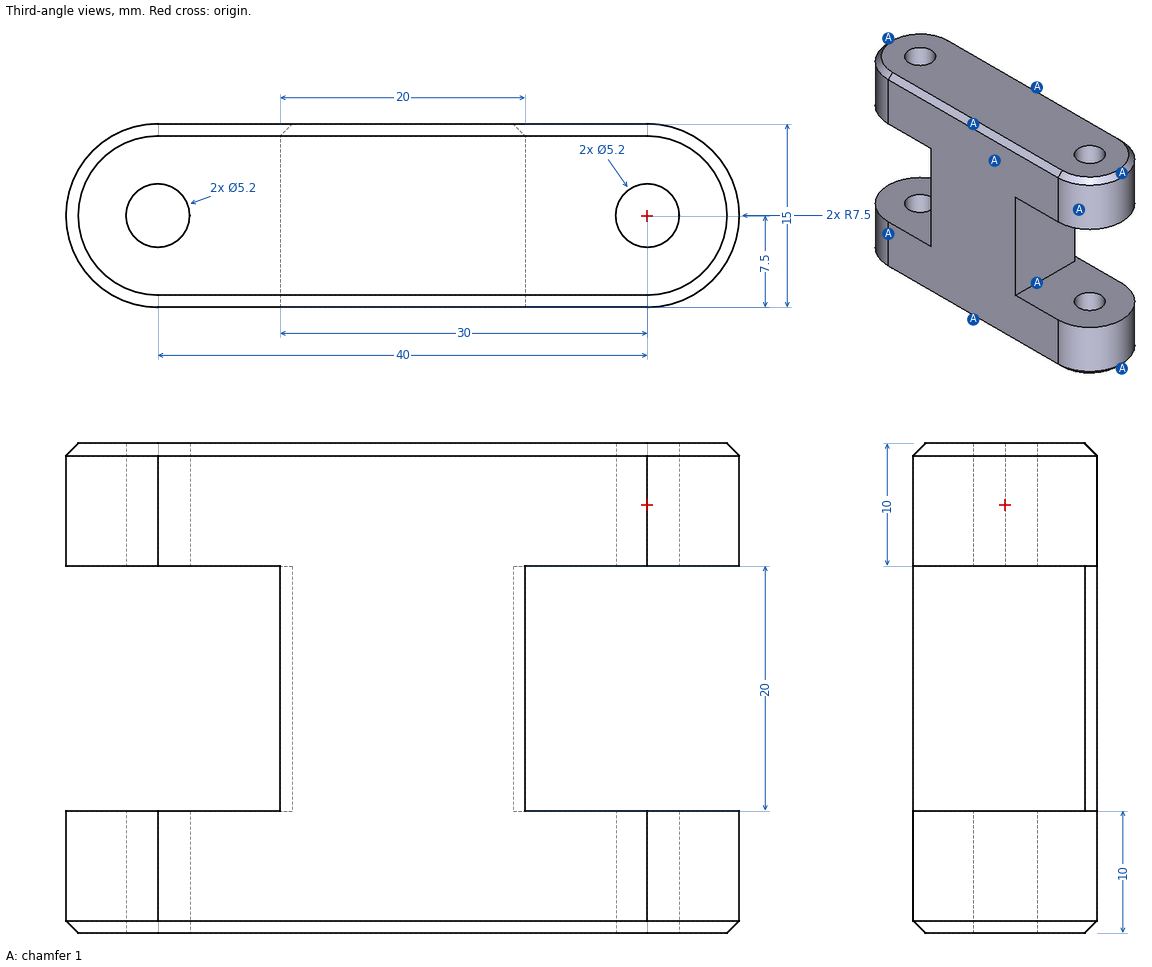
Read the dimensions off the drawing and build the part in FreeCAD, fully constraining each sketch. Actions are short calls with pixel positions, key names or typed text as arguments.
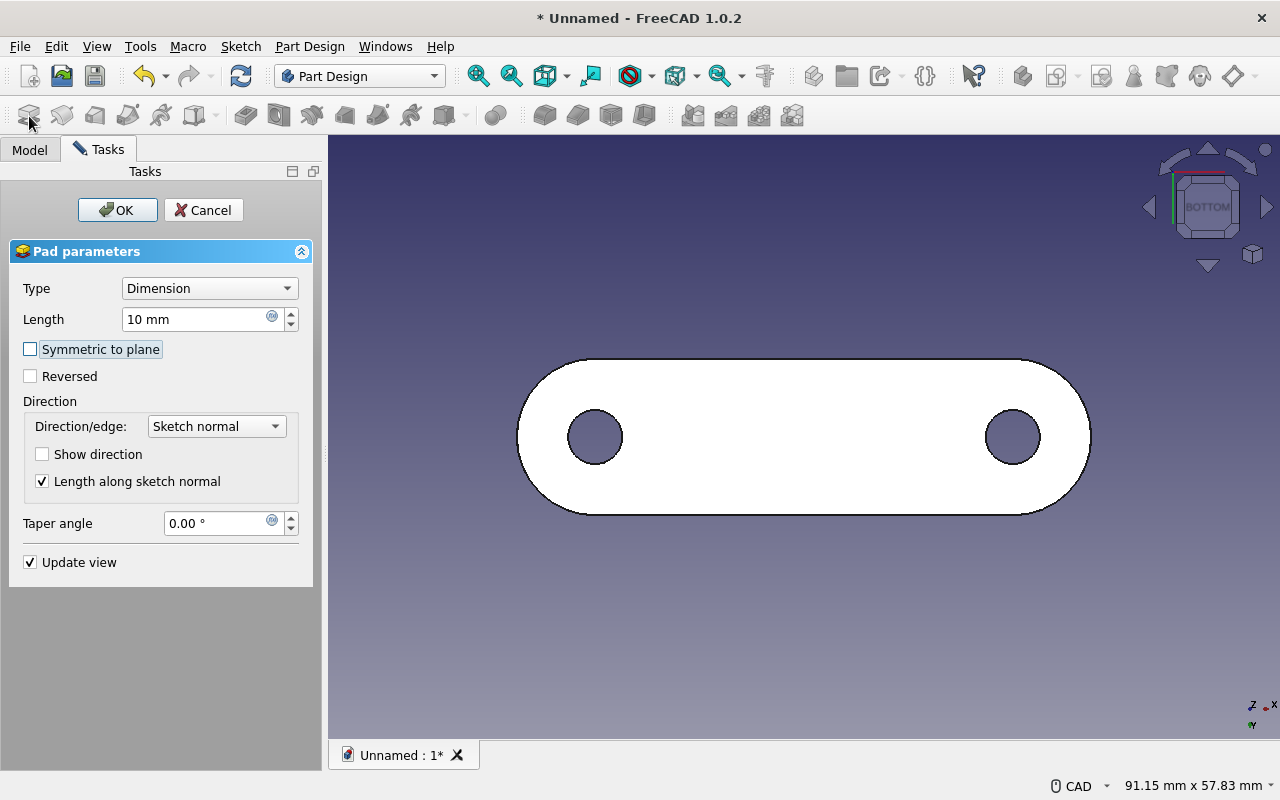
click(118, 210)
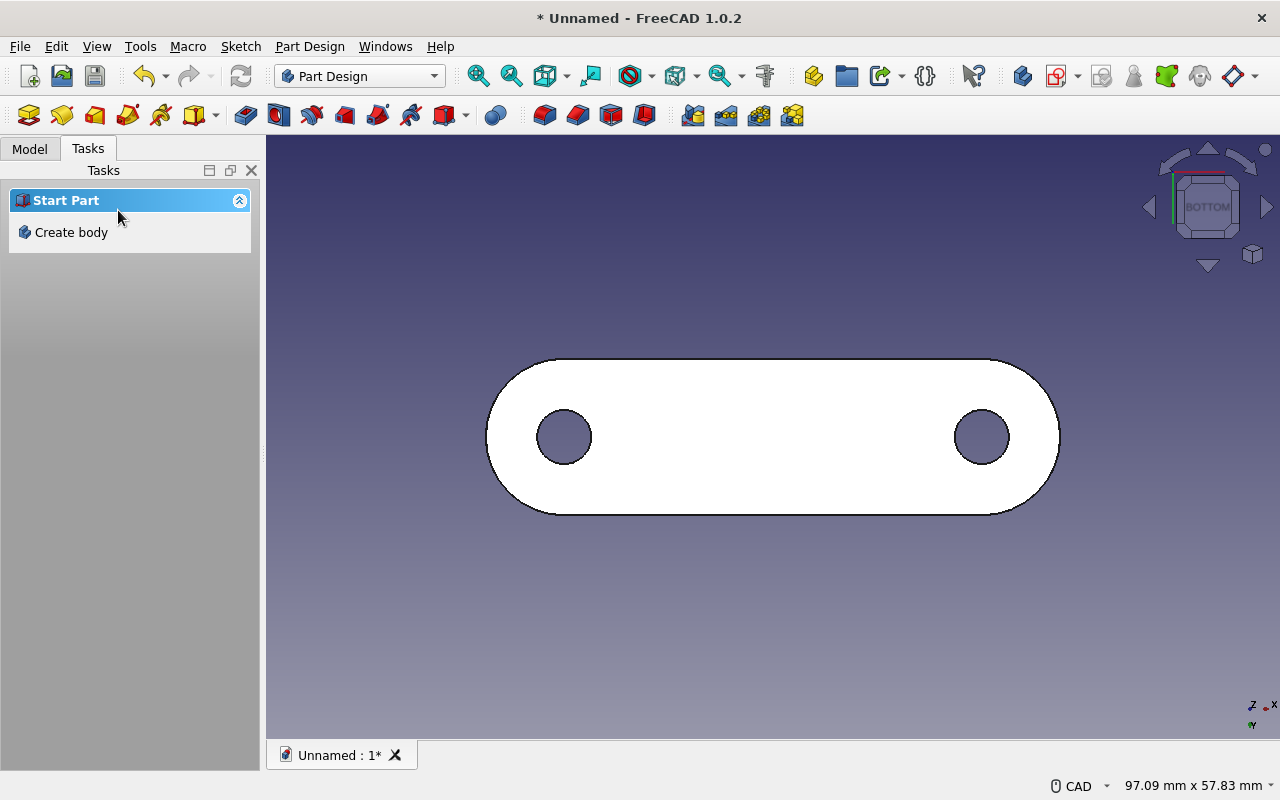
click(1060, 436)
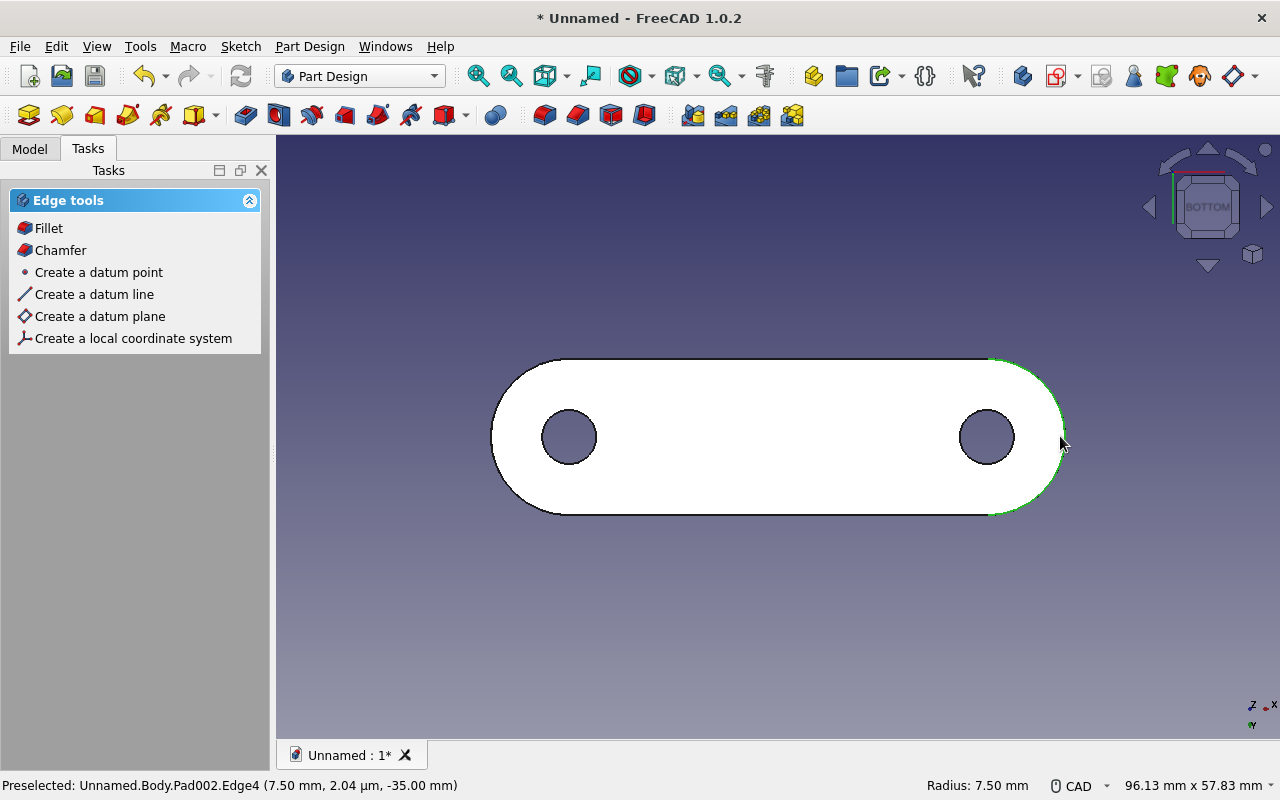
click(491, 436, ctrl)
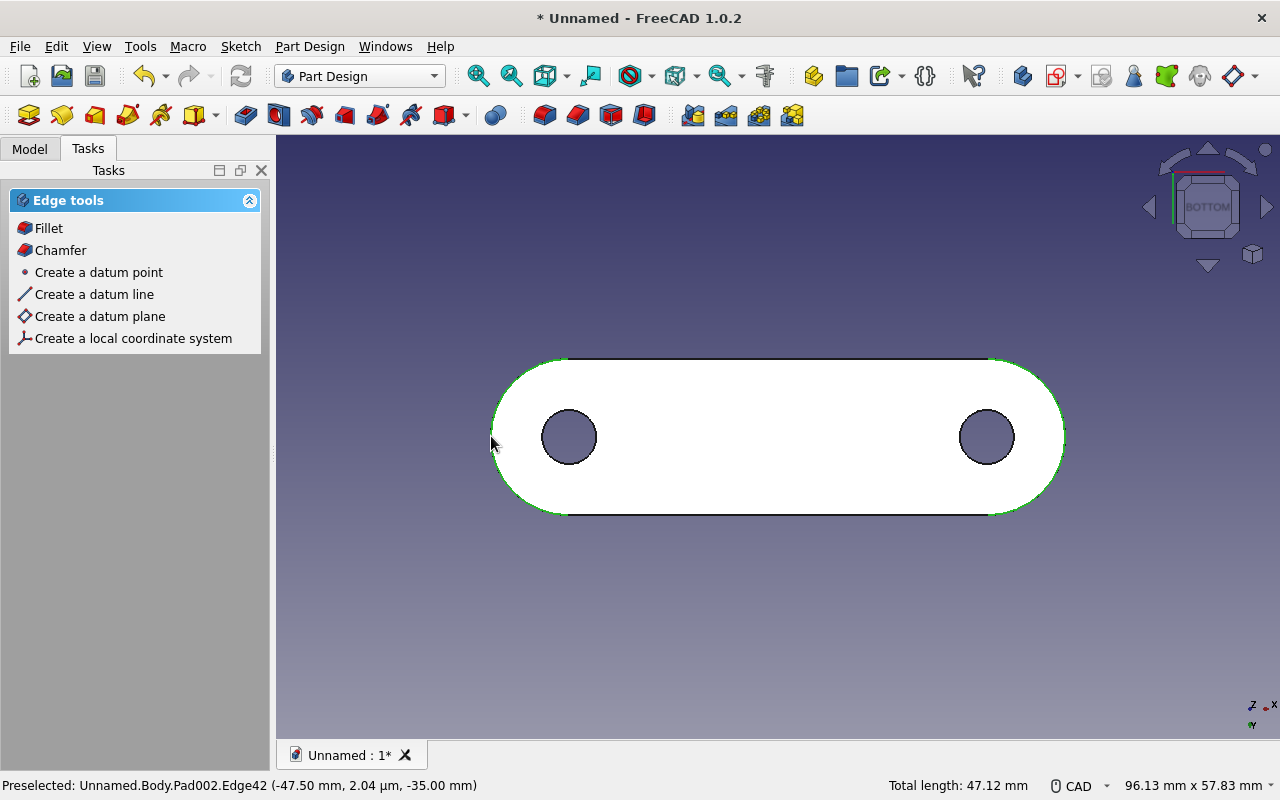
click(778, 514, ctrl)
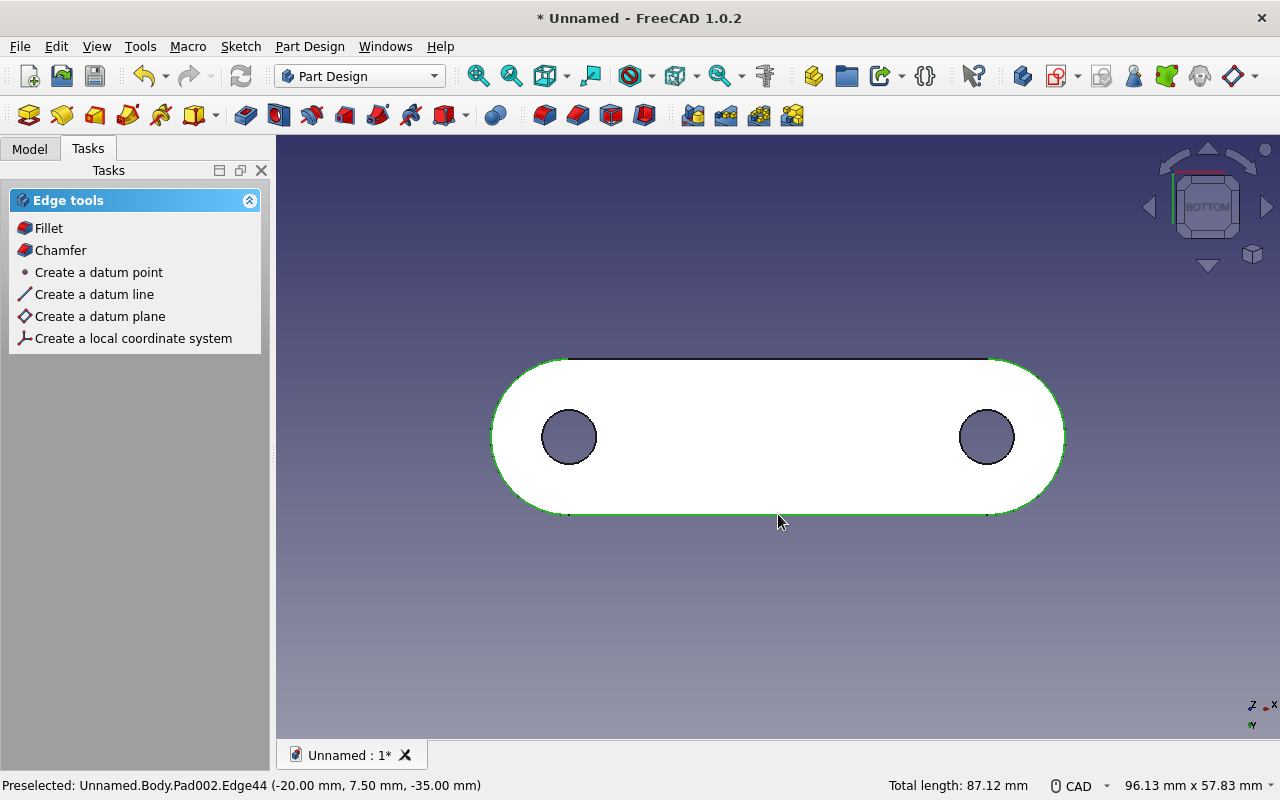
key(0)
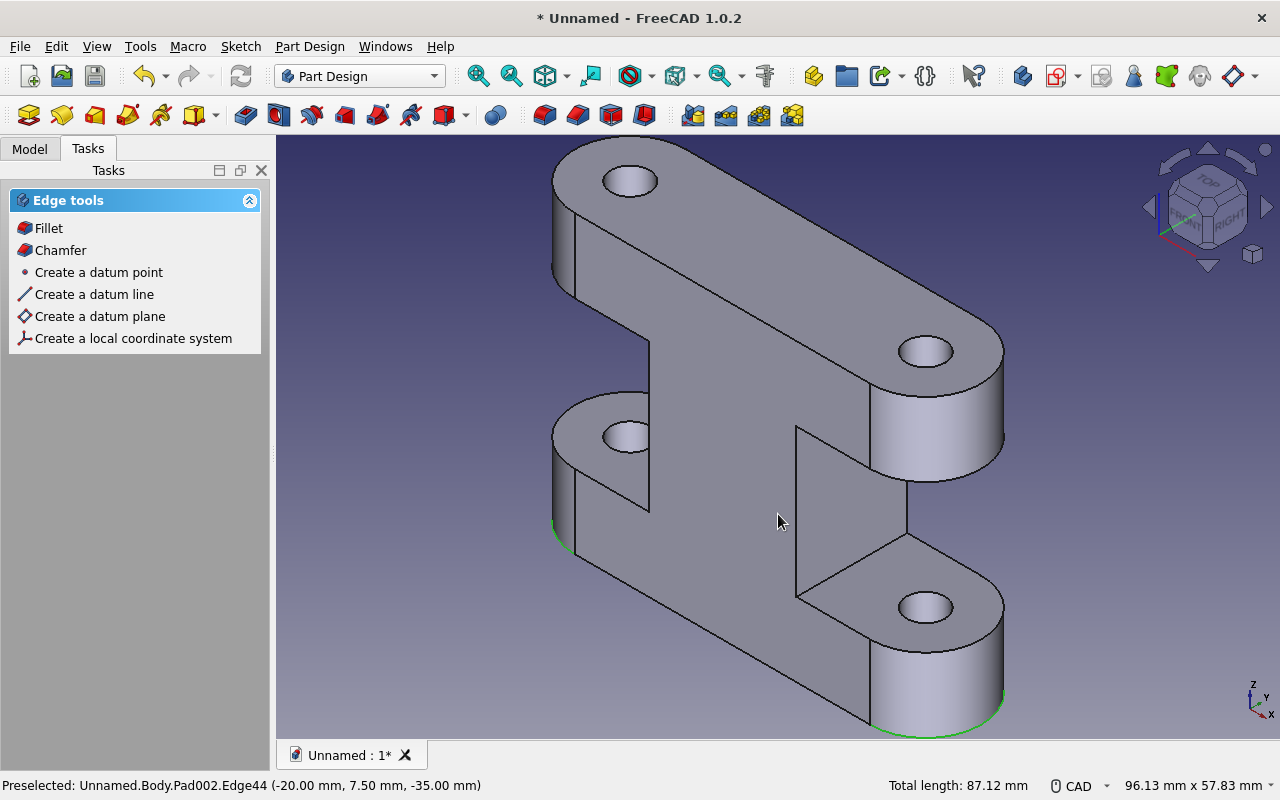
key(v)
key(f)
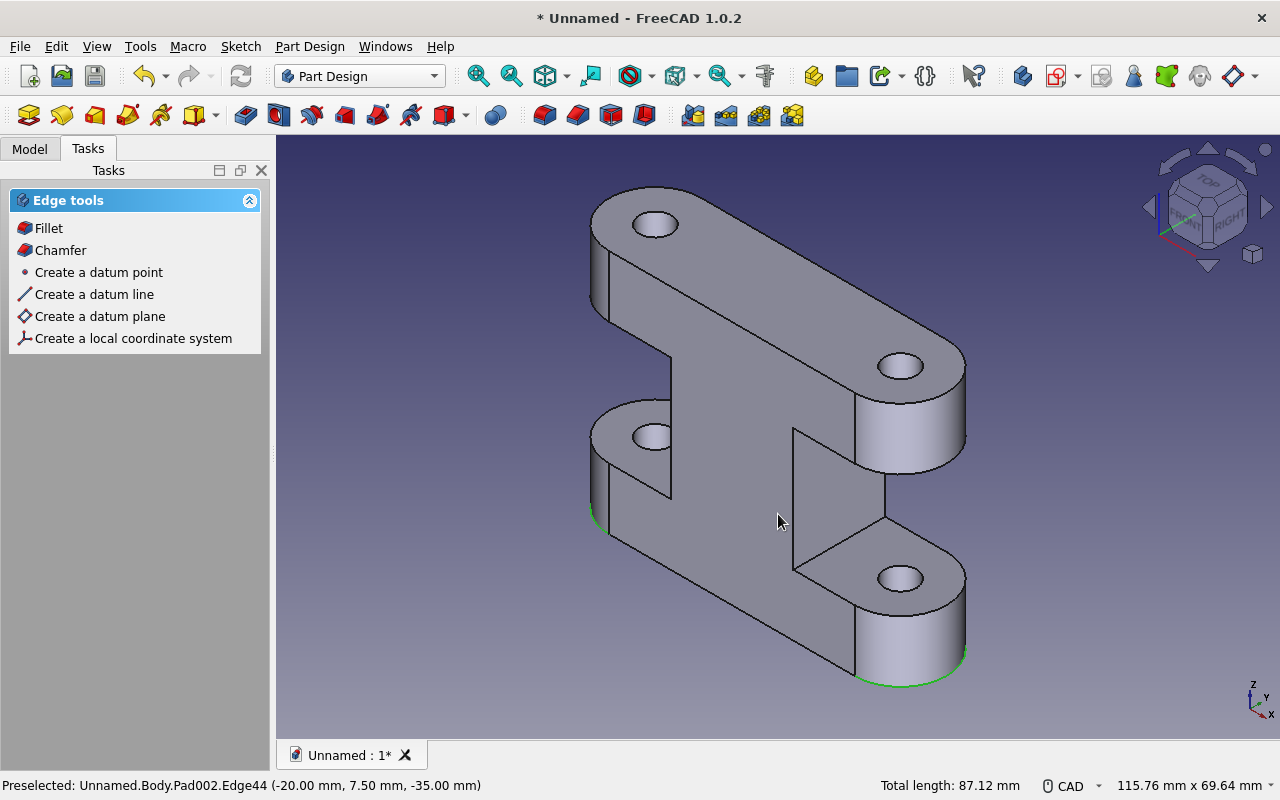
click(591, 229, ctrl)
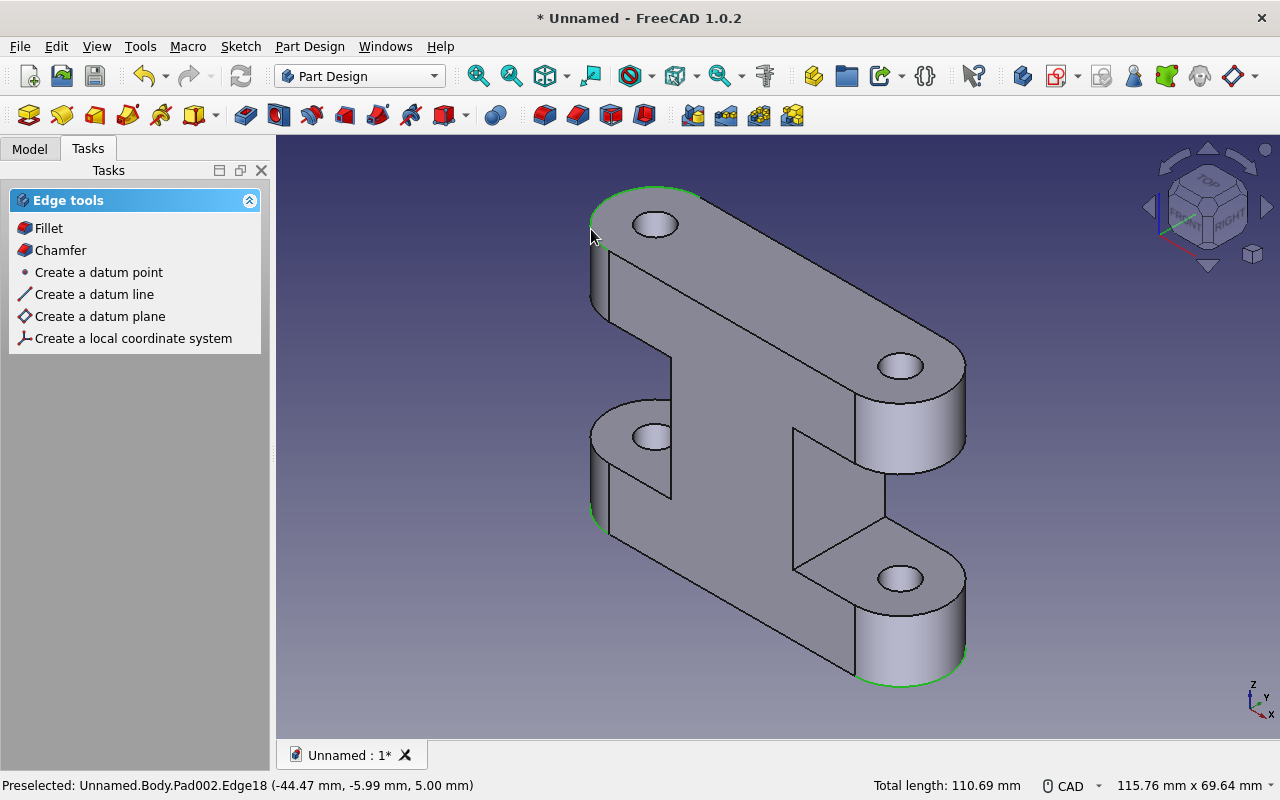
click(732, 321, ctrl)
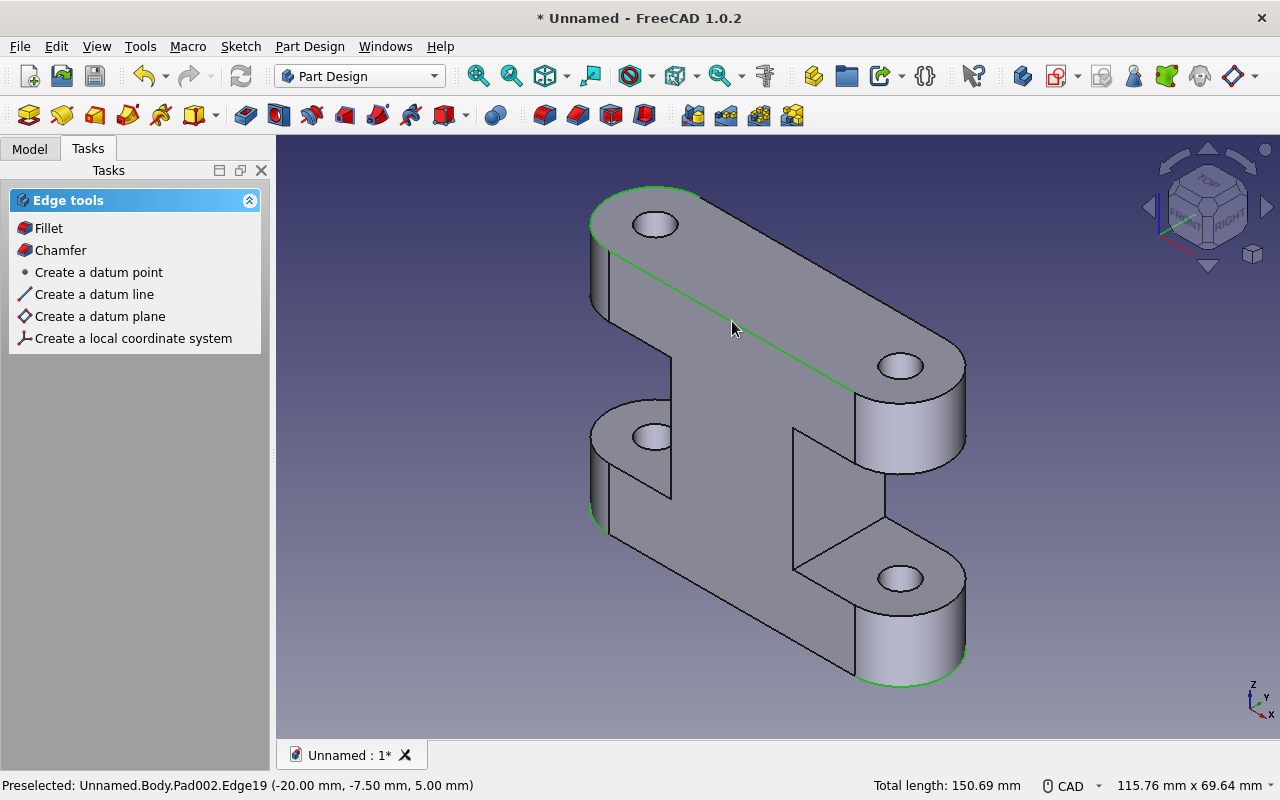
click(947, 392, ctrl)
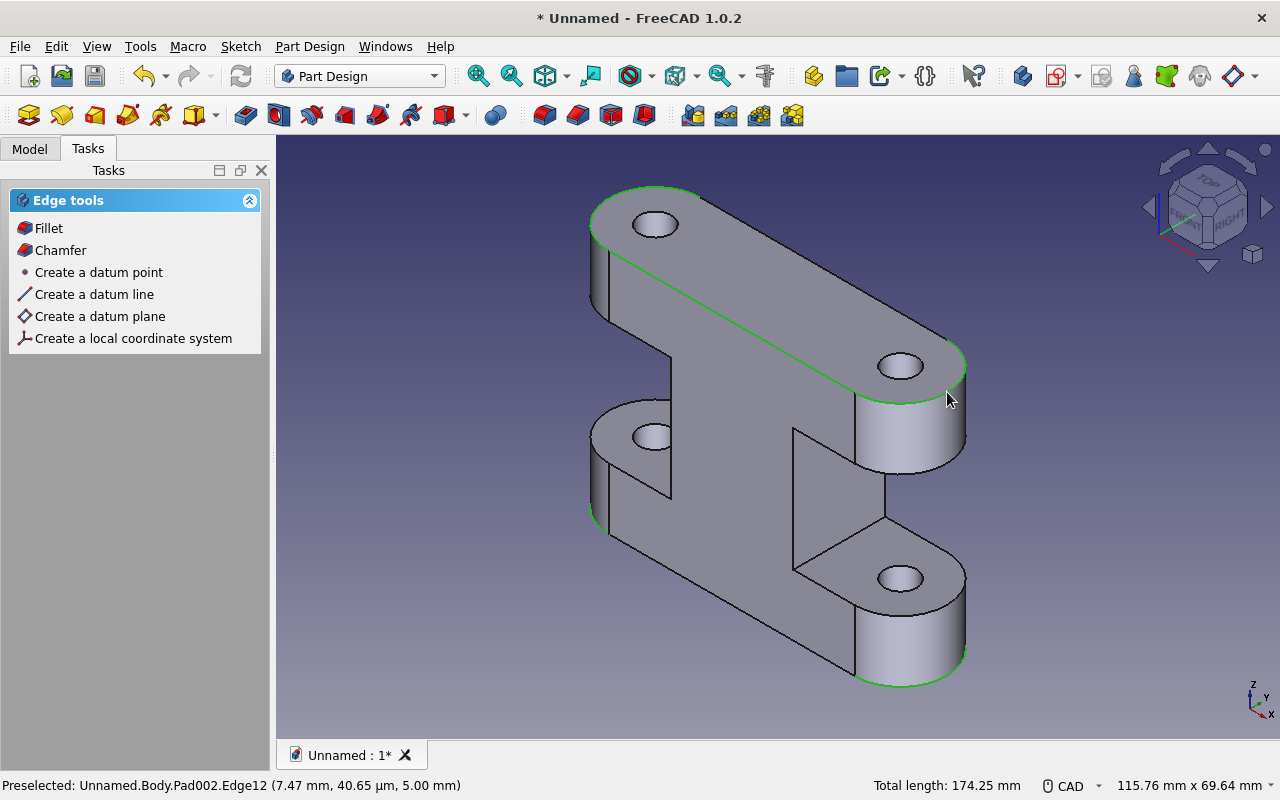
key(2)